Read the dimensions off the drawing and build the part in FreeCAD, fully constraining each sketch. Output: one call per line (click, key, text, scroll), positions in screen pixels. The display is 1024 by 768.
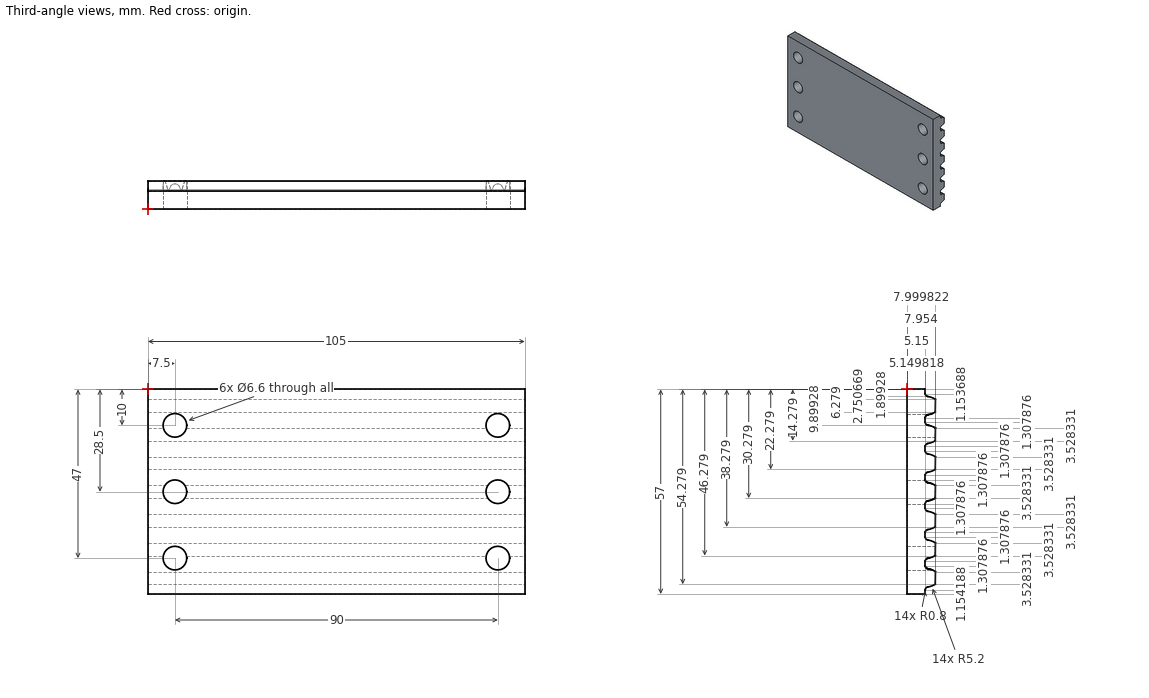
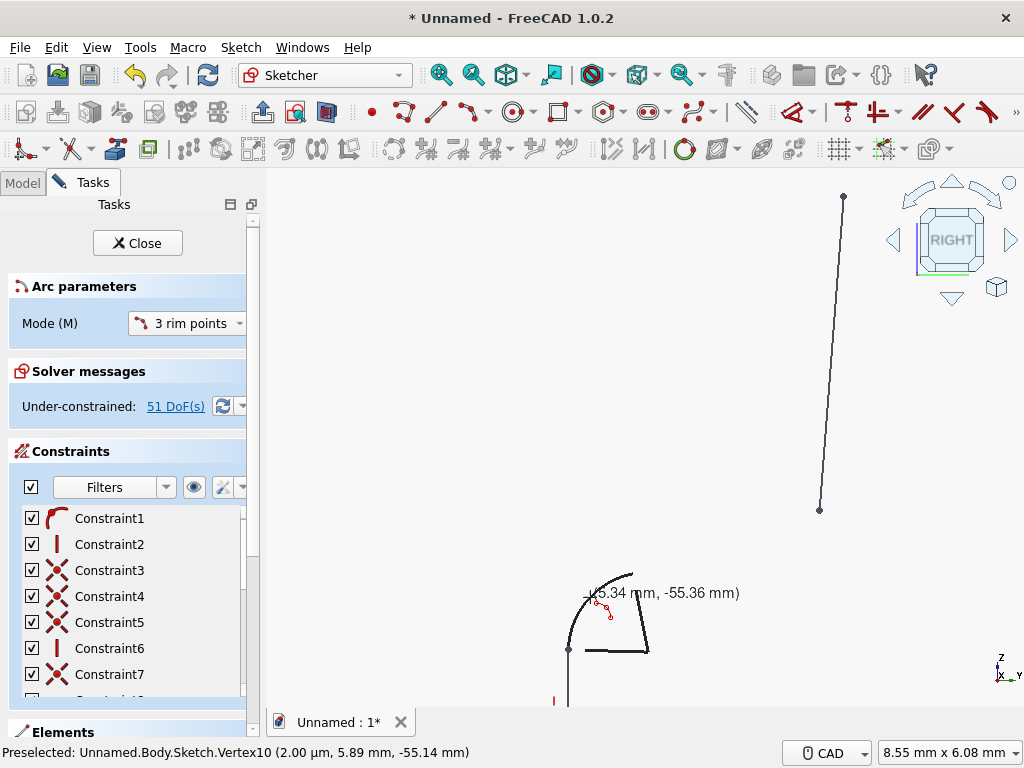
click(590, 595)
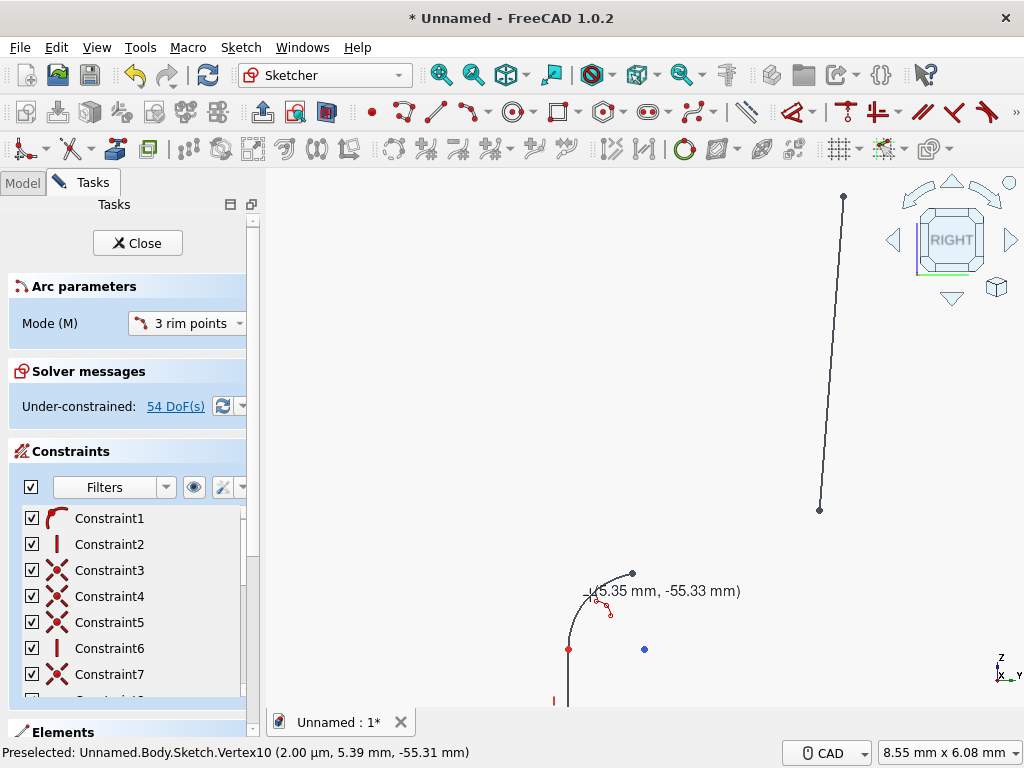
scroll(585, 616, down, 13)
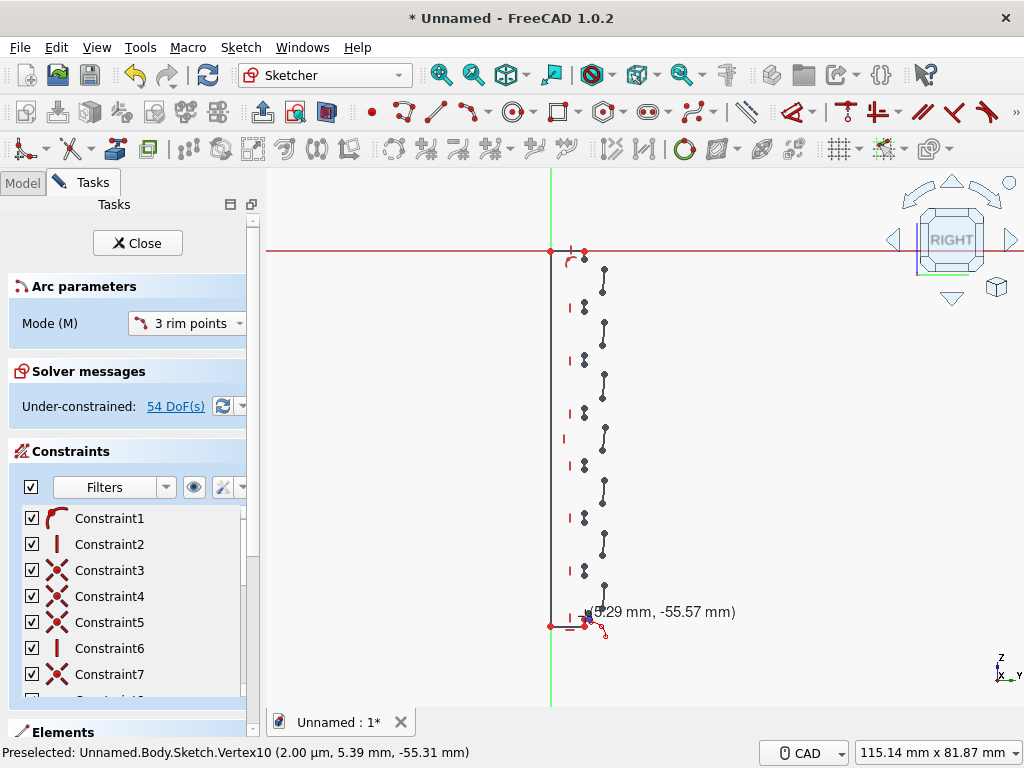
scroll(589, 613, up, 6)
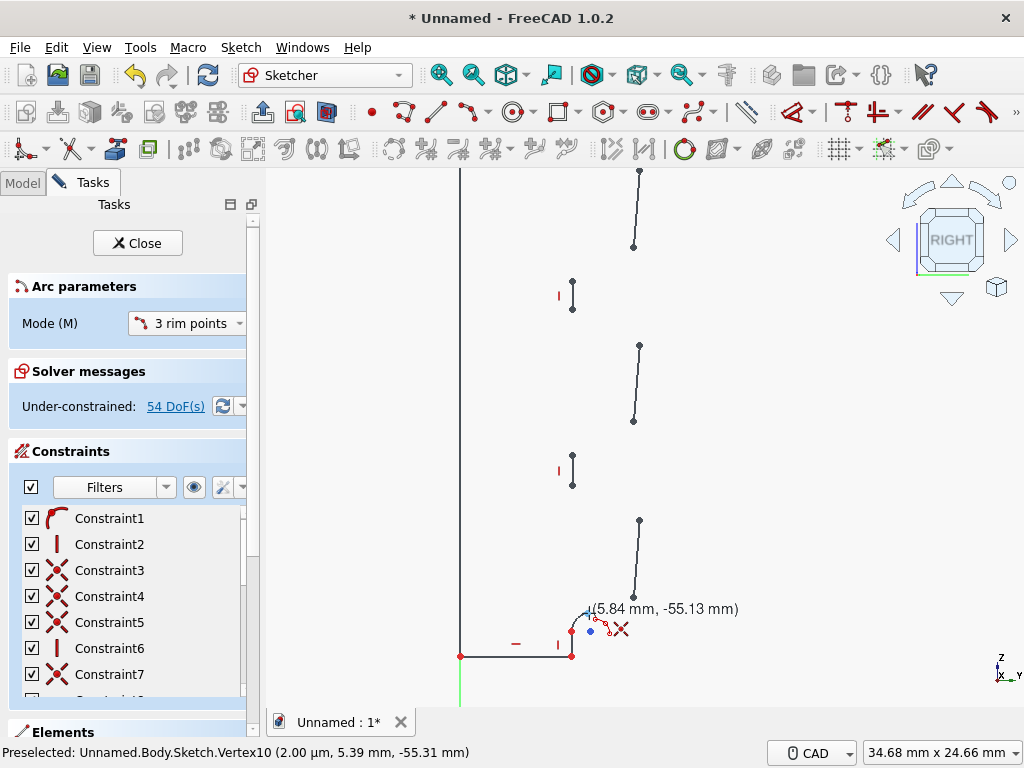
click(588, 613)
click(634, 598)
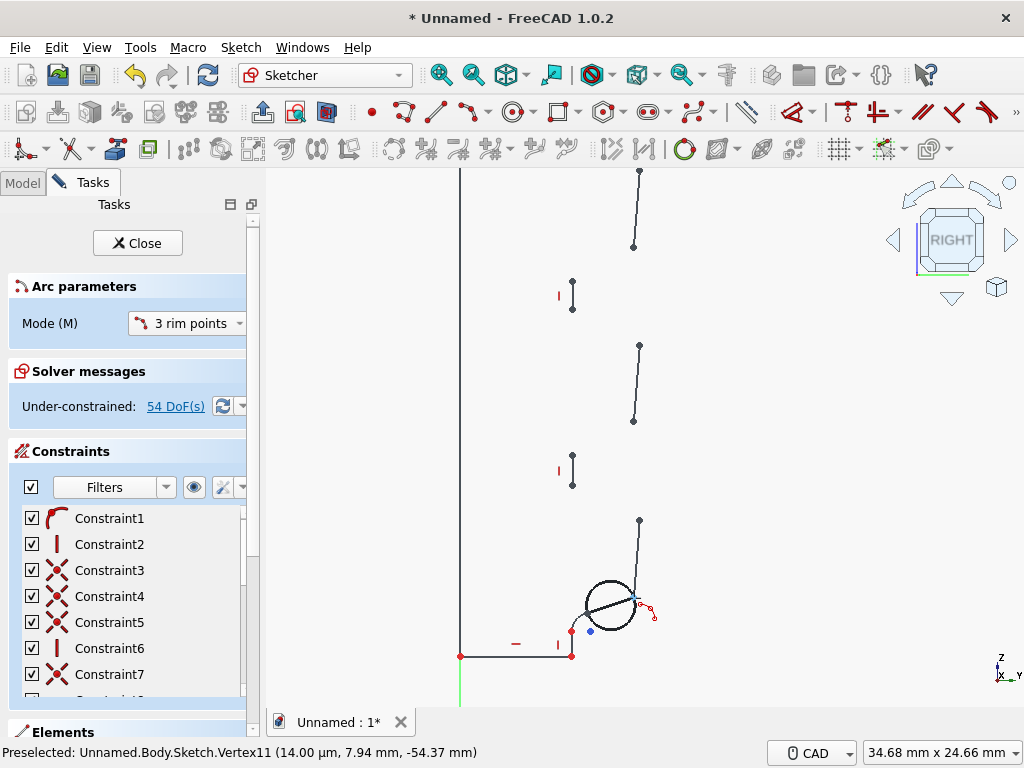
scroll(612, 607, up, 9)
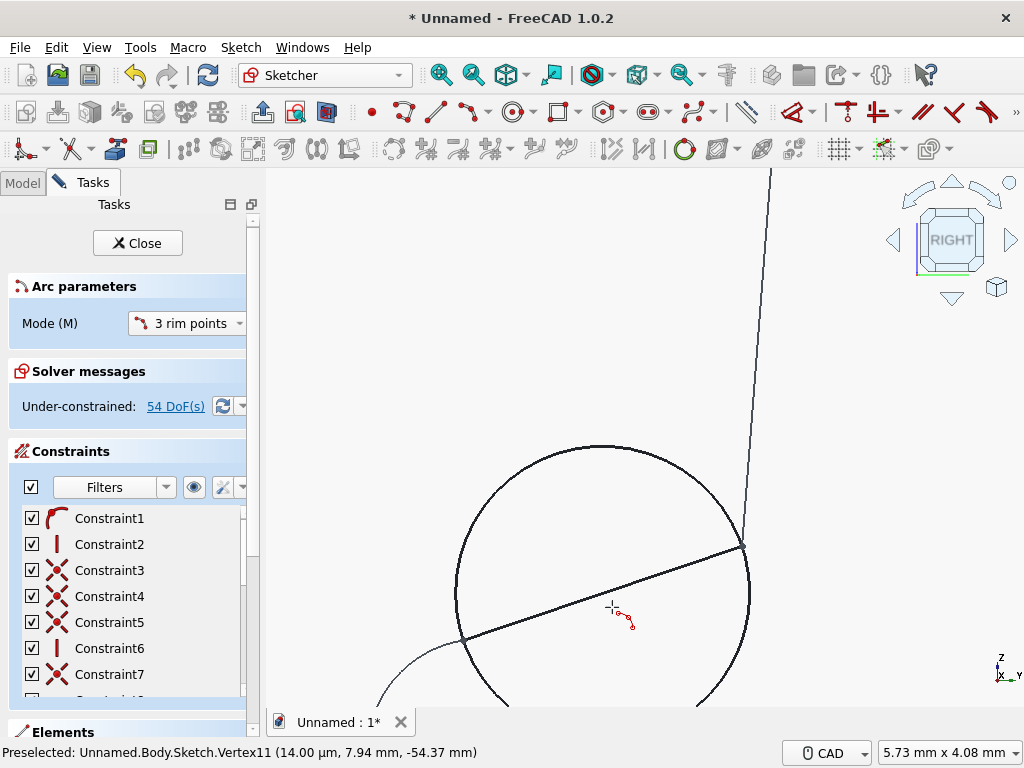
click(610, 601)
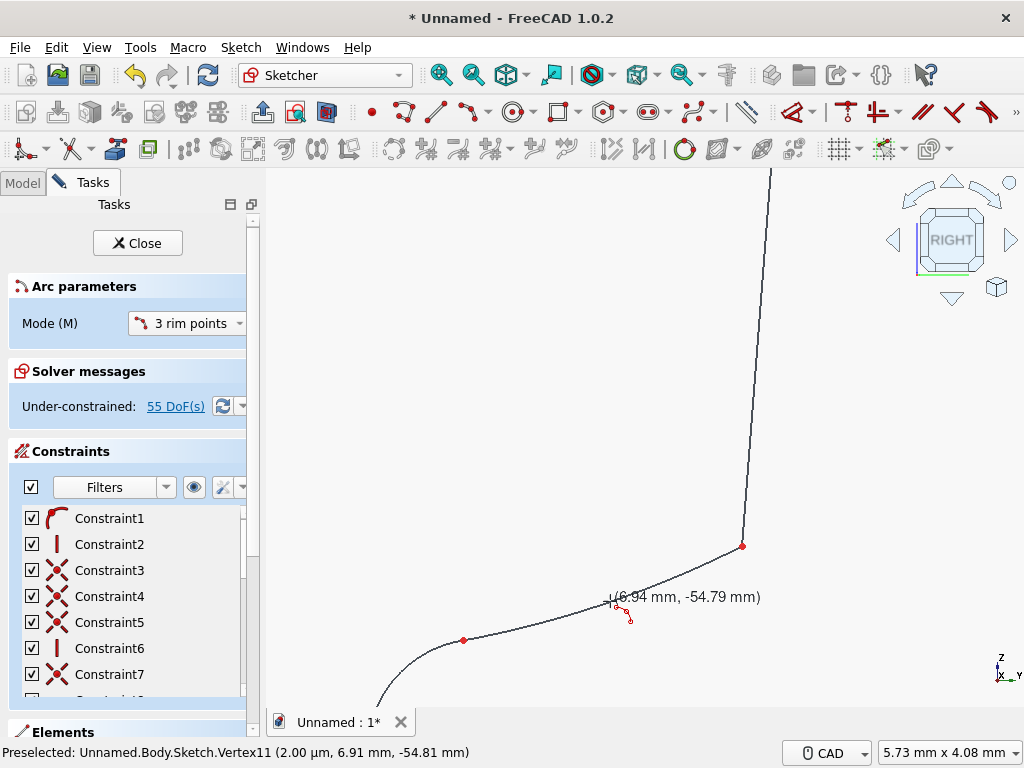
scroll(595, 611, down, 15)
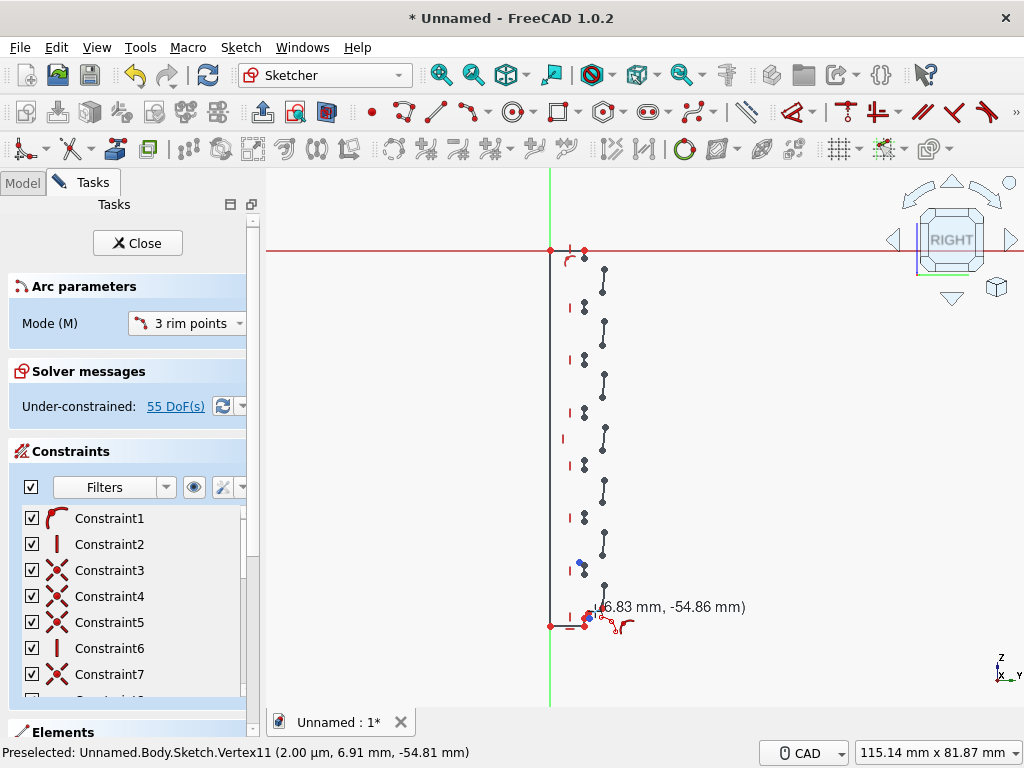
scroll(603, 585, up, 2)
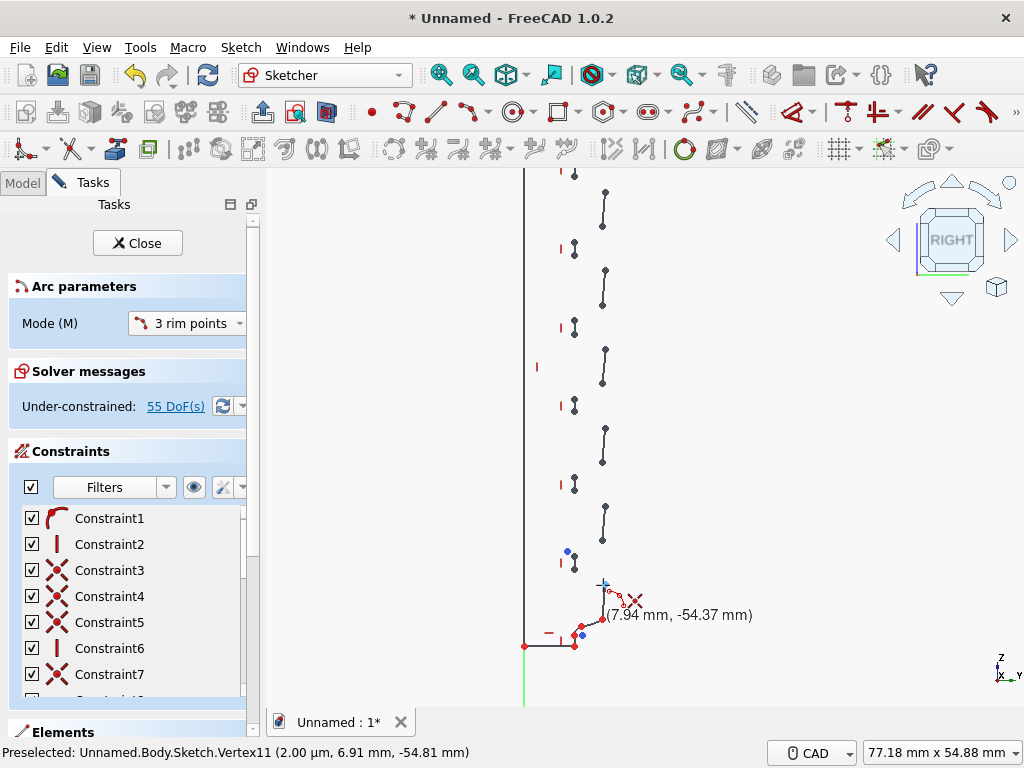
click(605, 585)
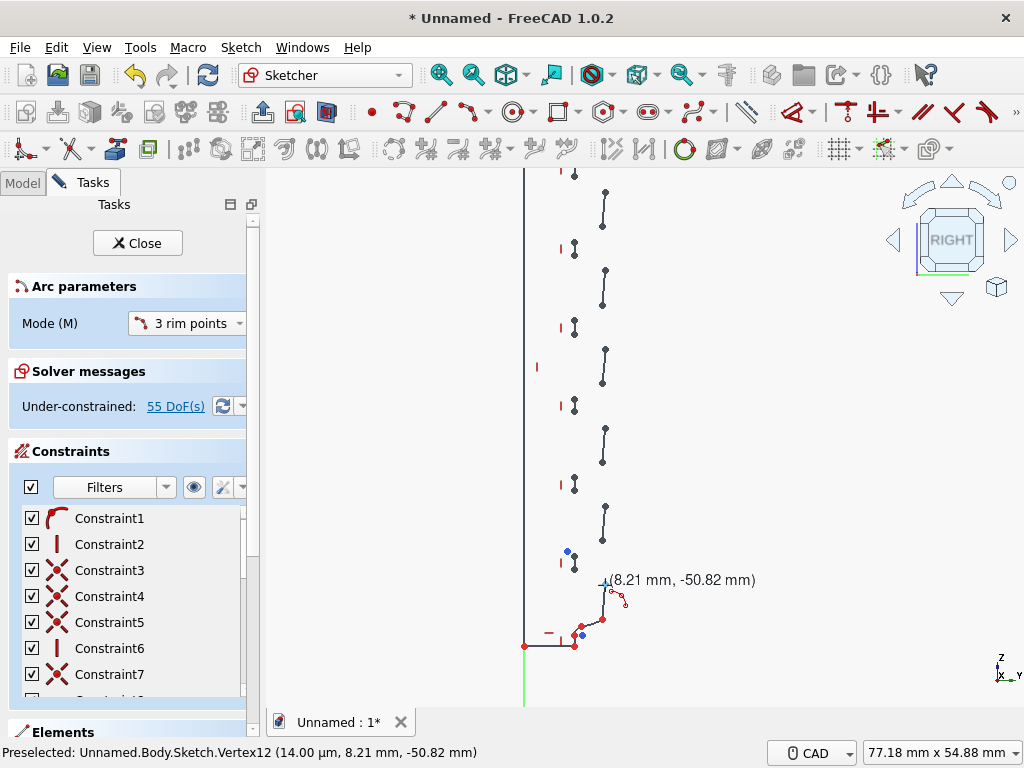
scroll(582, 576, up, 5)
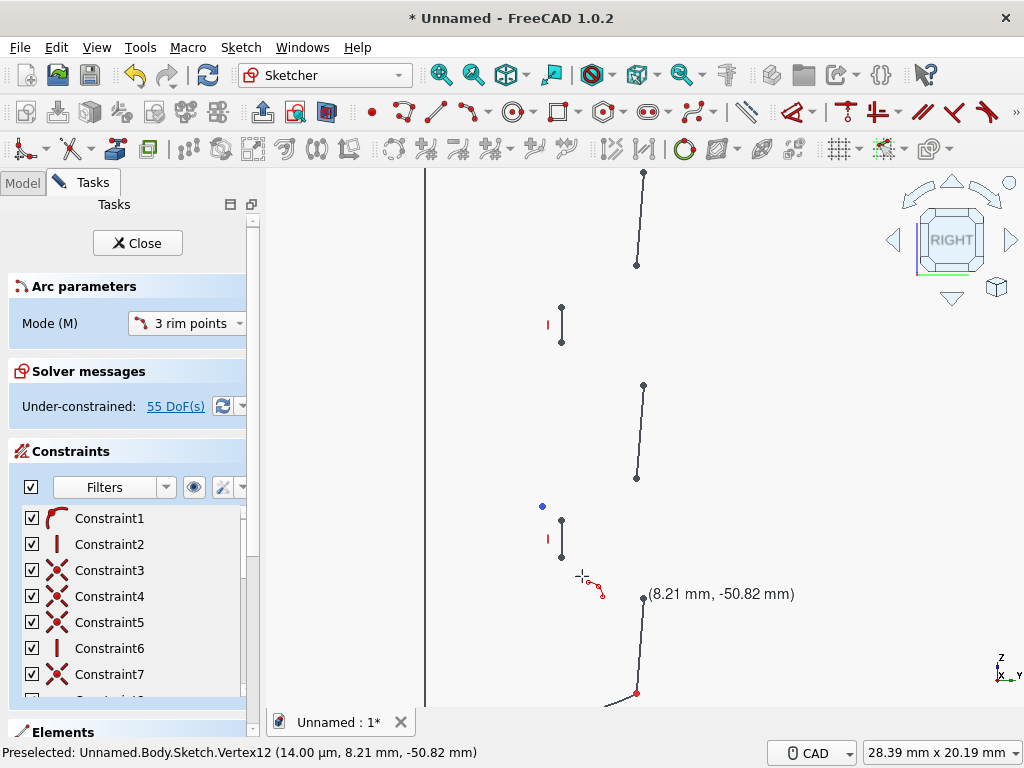
click(581, 576)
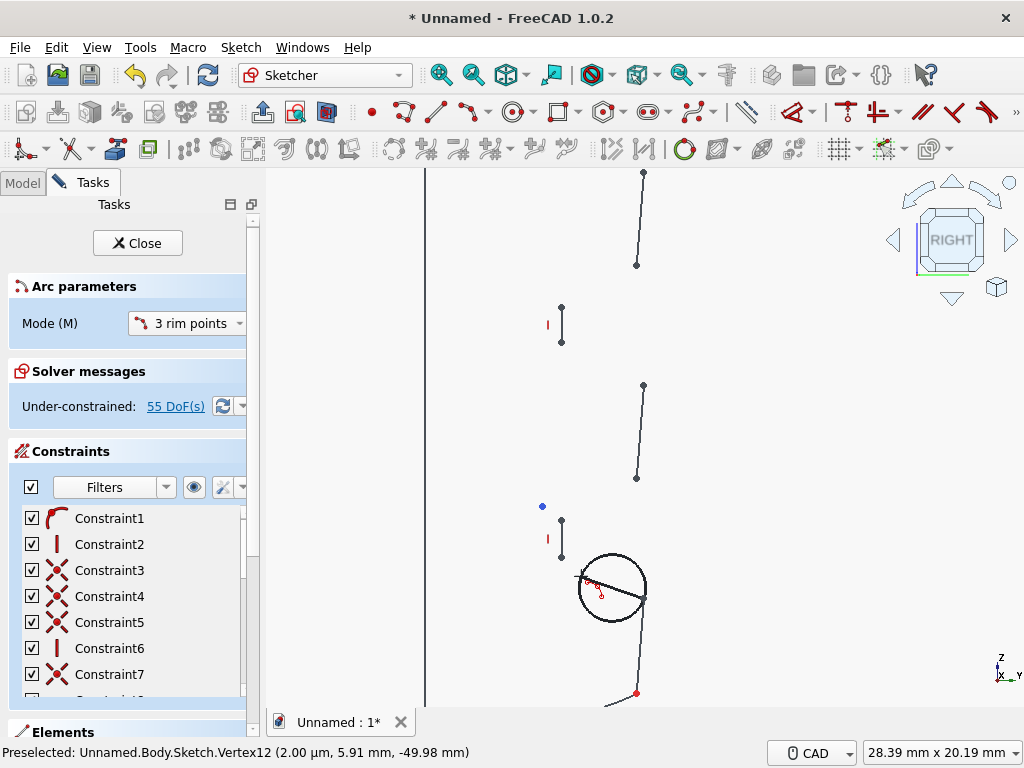
scroll(611, 583, up, 8)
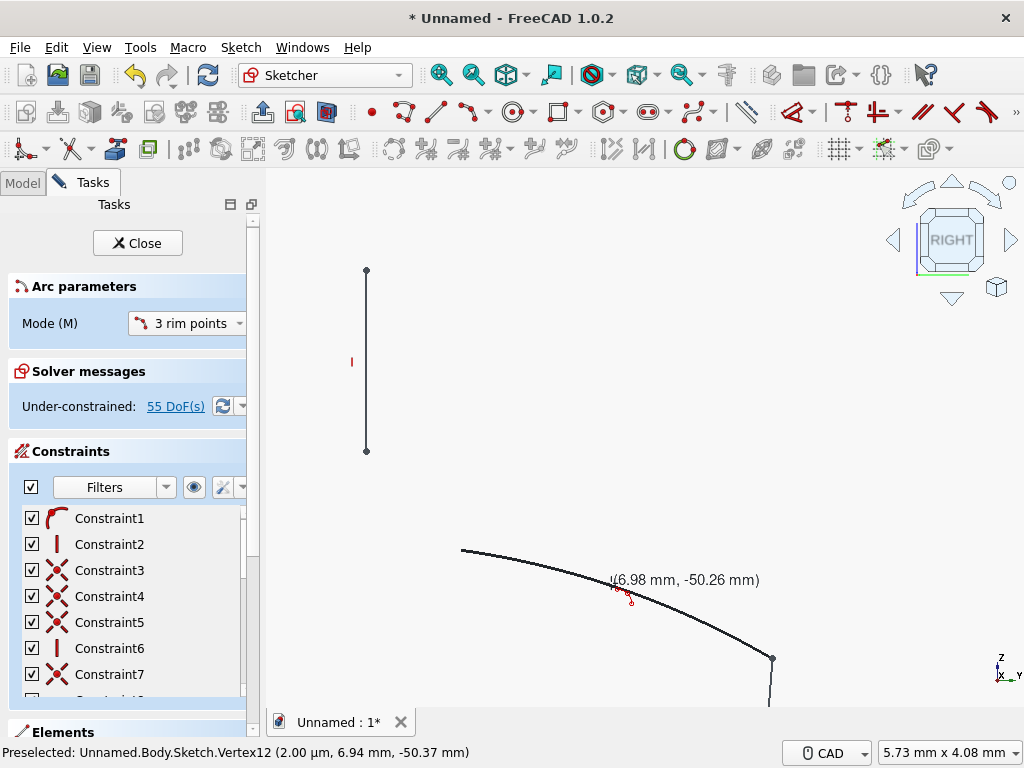
click(608, 581)